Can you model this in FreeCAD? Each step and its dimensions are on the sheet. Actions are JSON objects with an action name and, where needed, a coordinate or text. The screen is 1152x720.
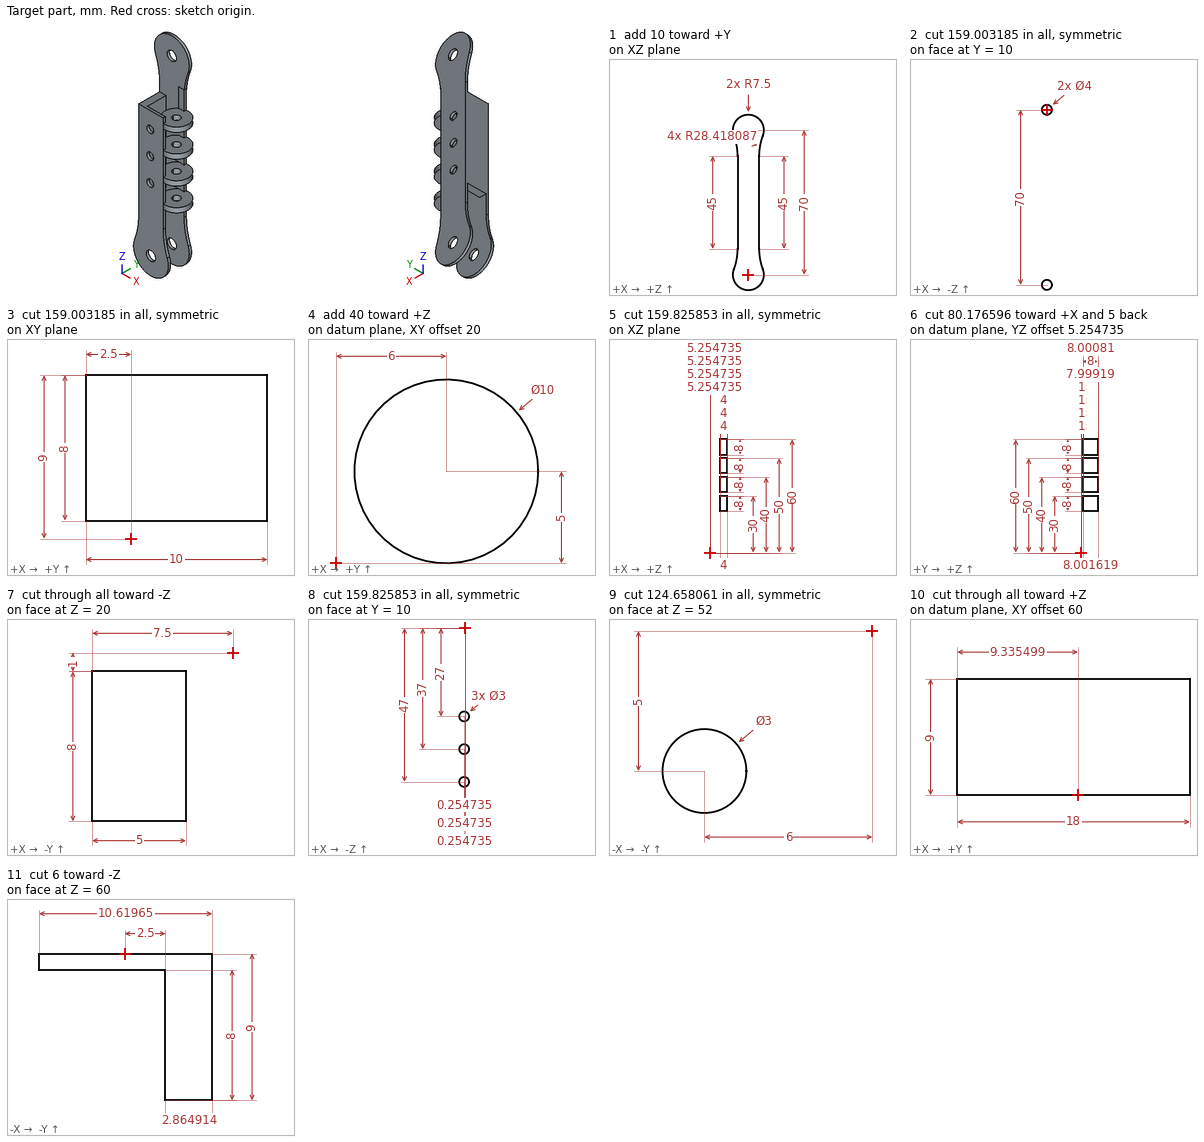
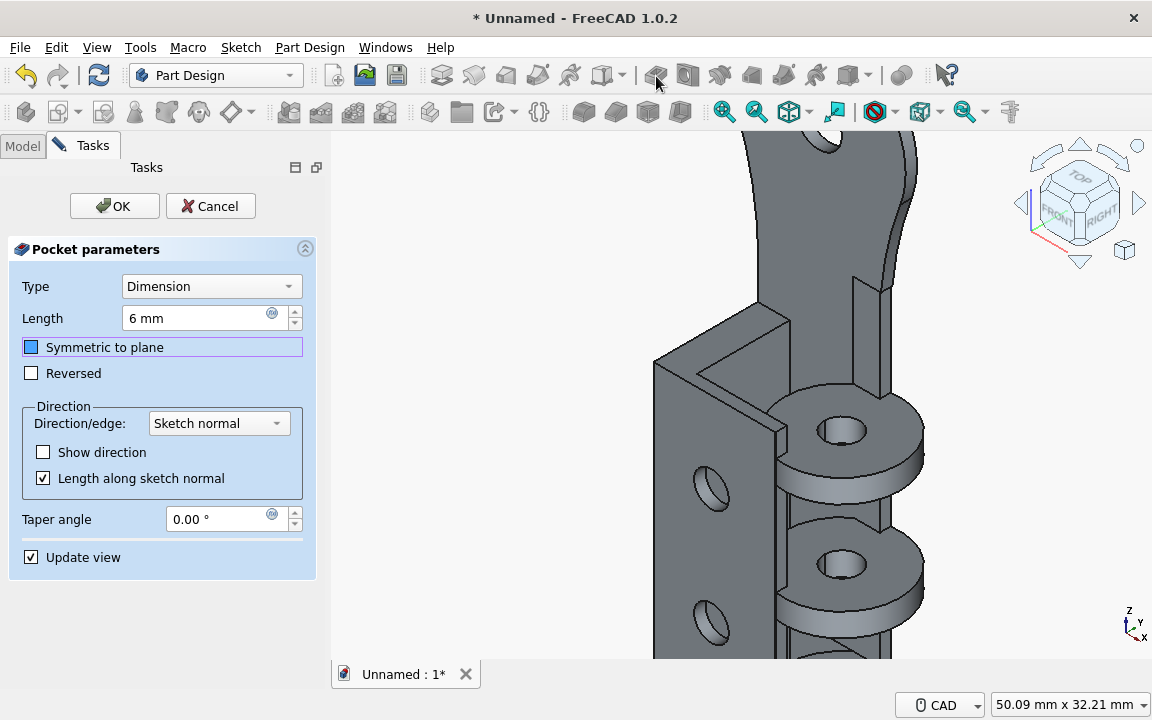
{"action": "left_click", "coordinate": [115, 206]}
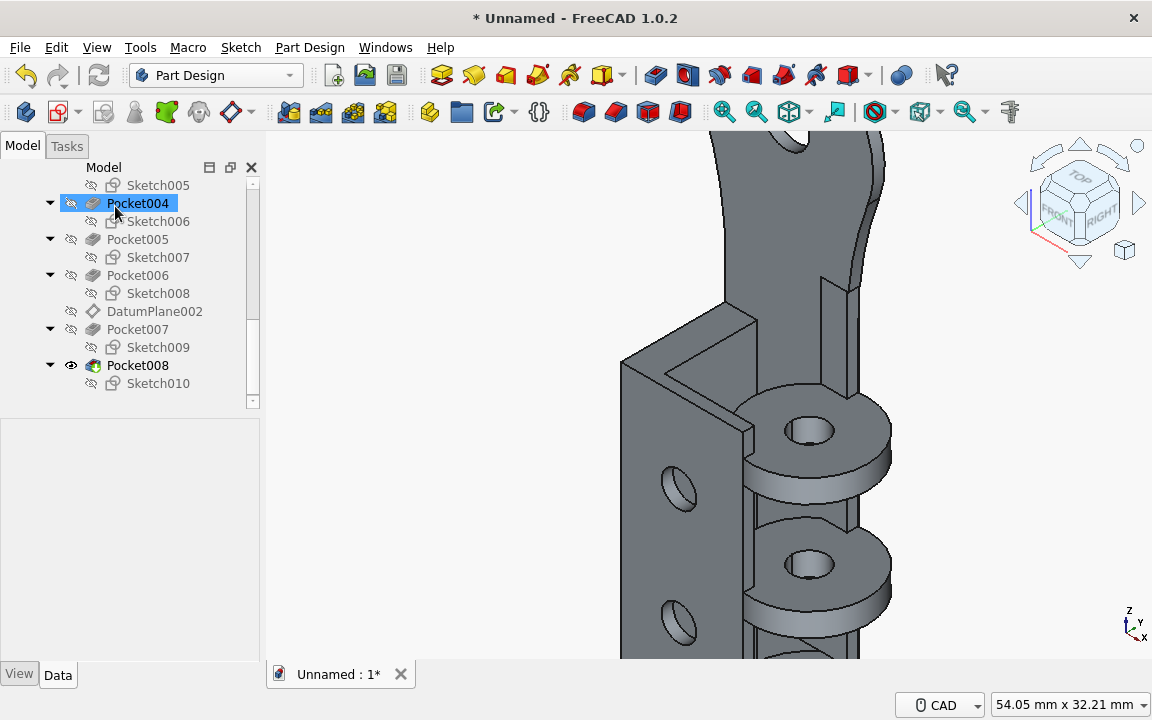
{"action": "left_click", "coordinate": [726, 112]}